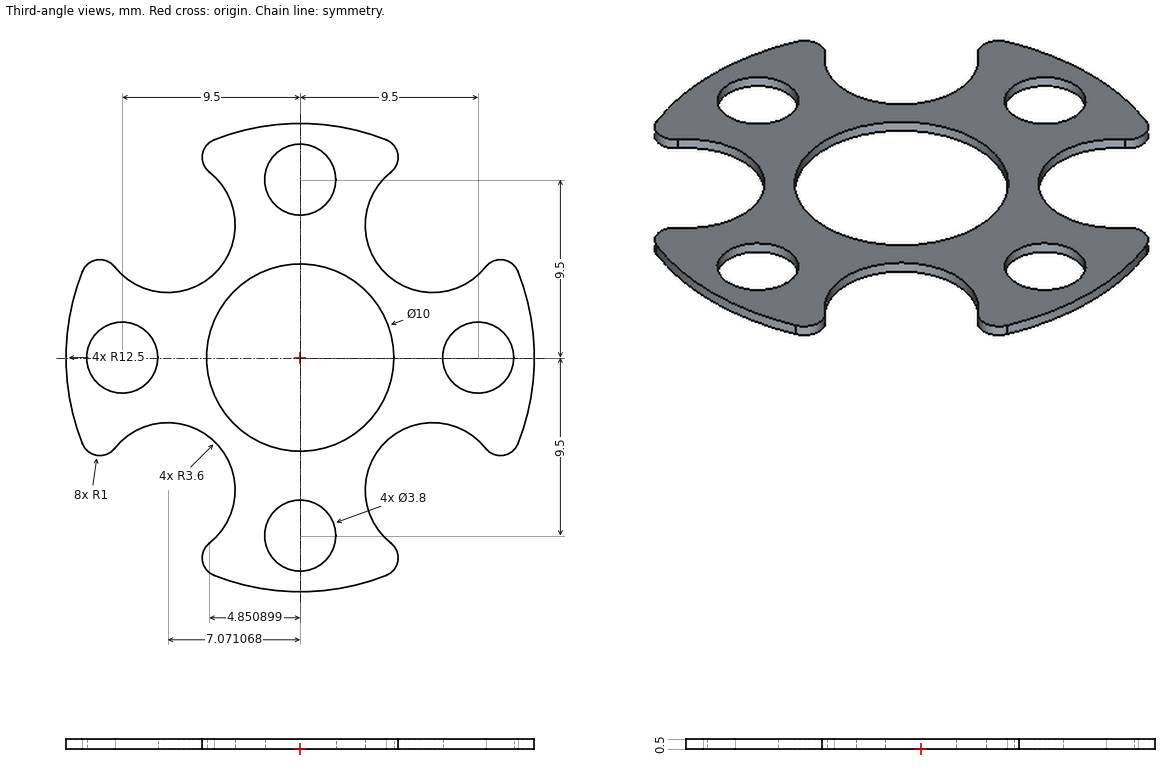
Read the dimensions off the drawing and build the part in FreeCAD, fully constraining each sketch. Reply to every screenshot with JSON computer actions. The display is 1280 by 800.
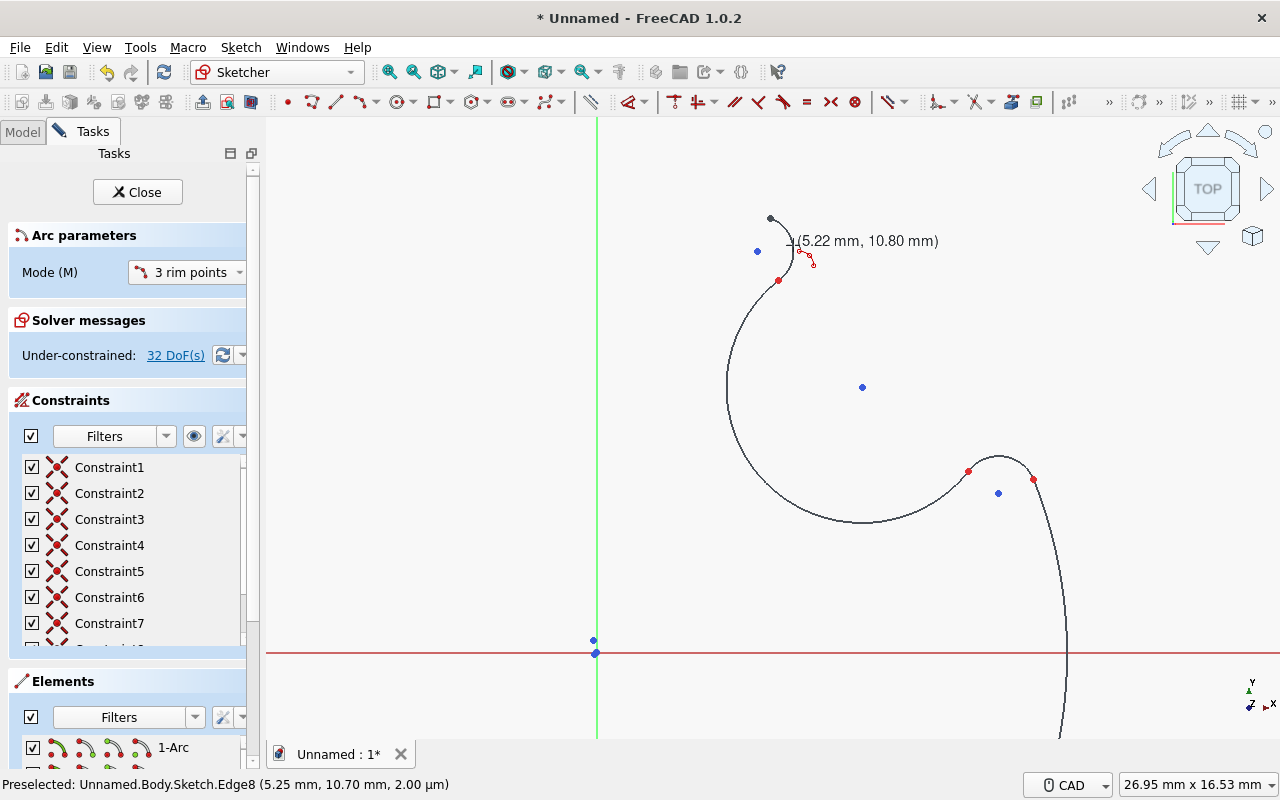
{"action": "left_click", "coordinate": [770, 218]}
{"action": "left_click", "coordinate": [423, 215]}
{"action": "left_click", "coordinate": [632, 184]}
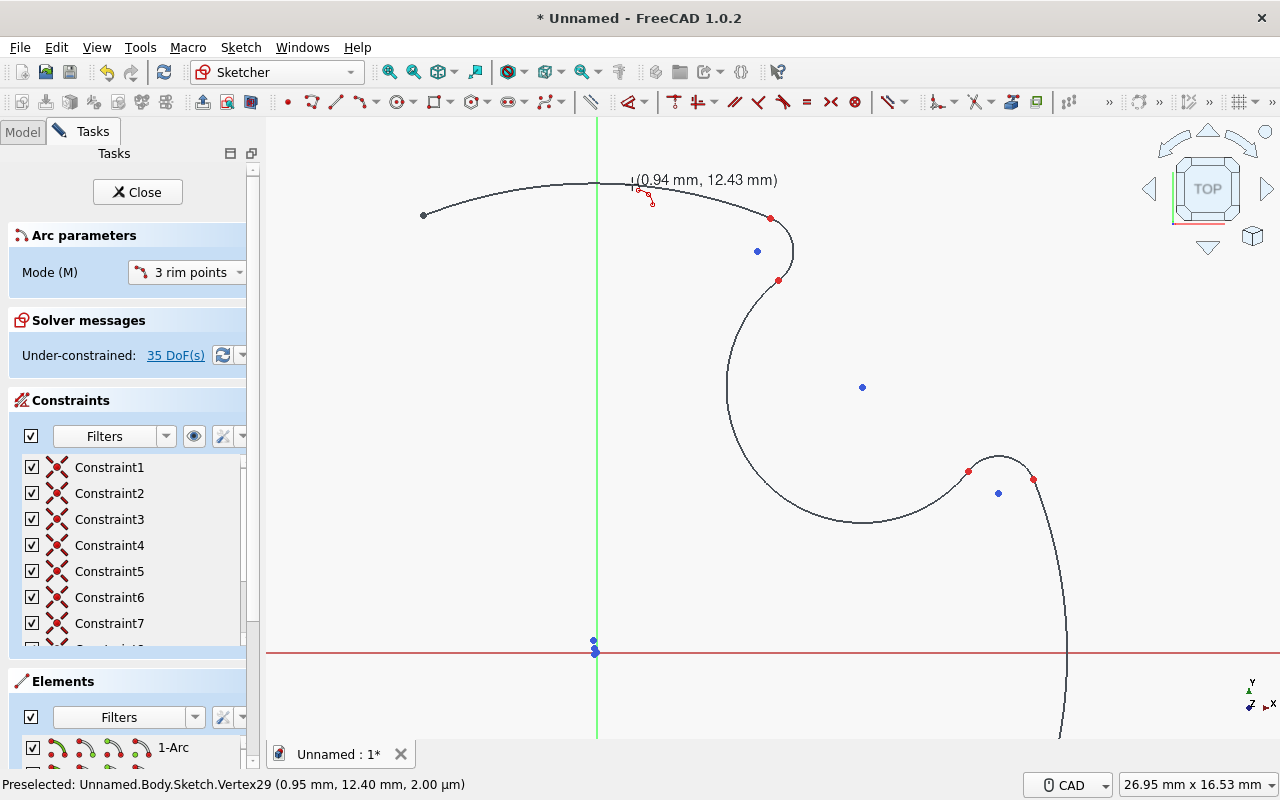
{"action": "left_click", "coordinate": [423, 216]}
{"action": "left_click", "coordinate": [414, 280]}
{"action": "left_click", "coordinate": [400, 245]}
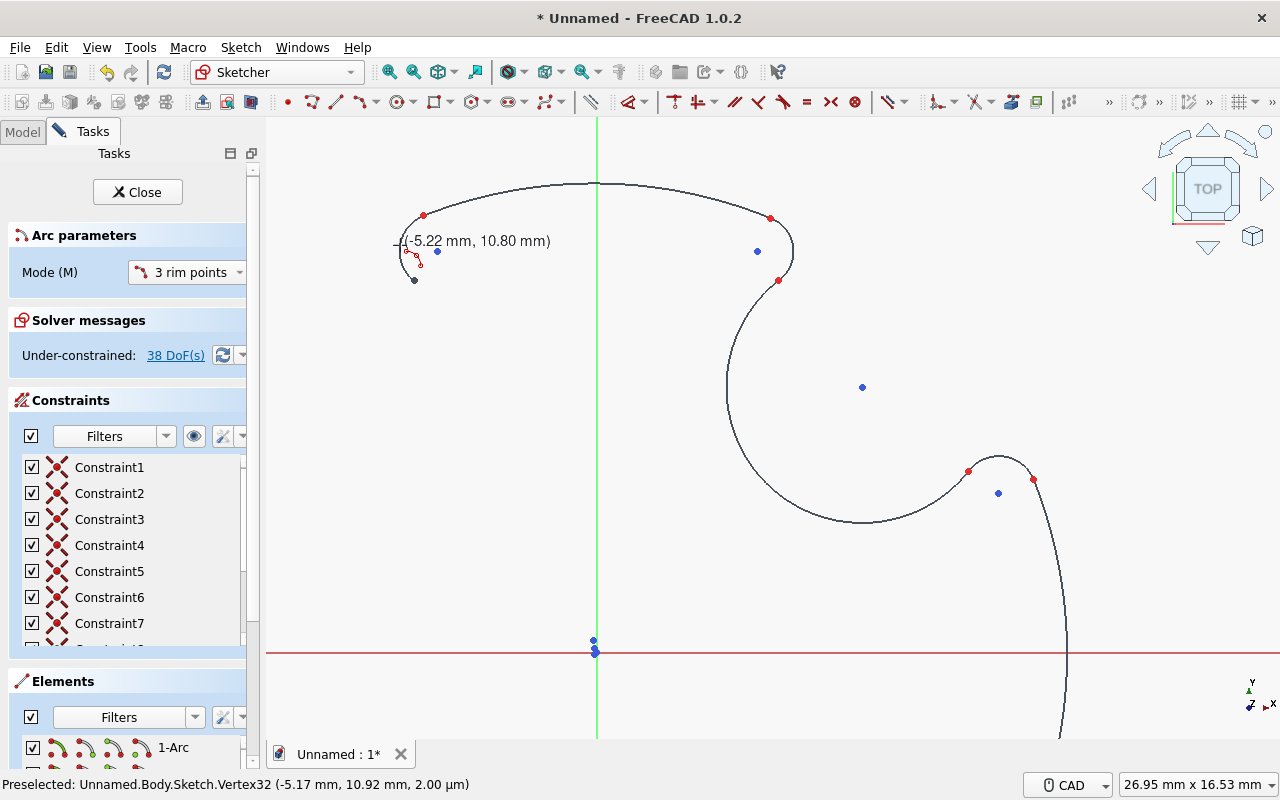
{"action": "left_click", "coordinate": [414, 281]}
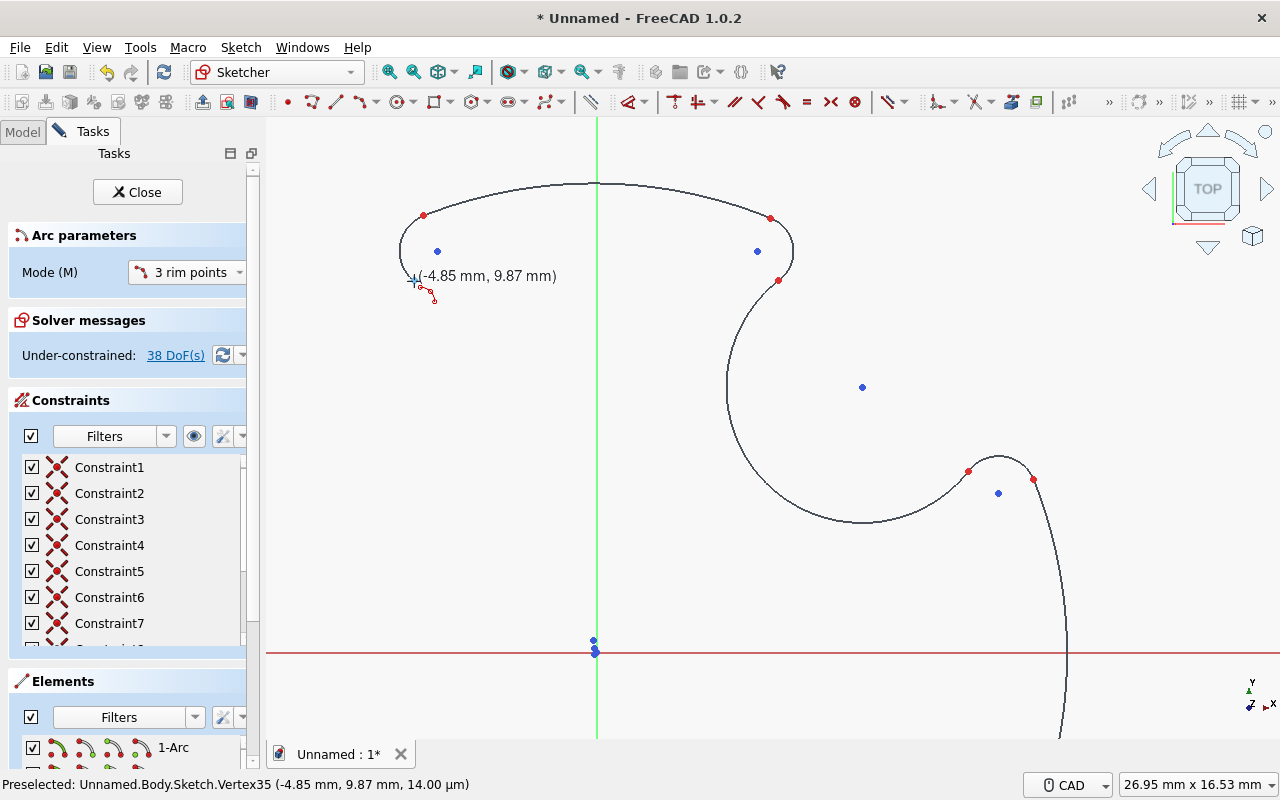
{"action": "scroll", "coordinate": [793, 245], "scroll_direction": "down", "scroll_amount": 4}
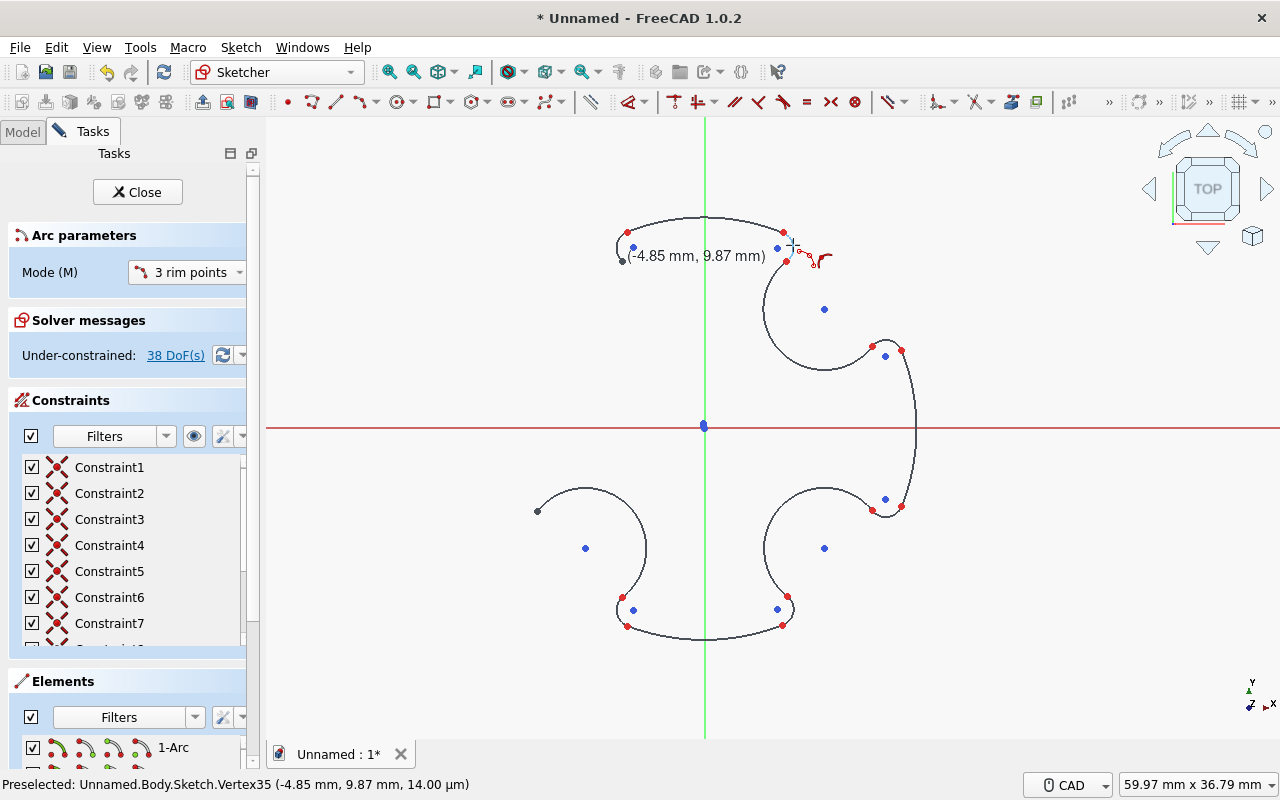
{"action": "left_click", "coordinate": [538, 346]}
{"action": "left_click", "coordinate": [628, 352]}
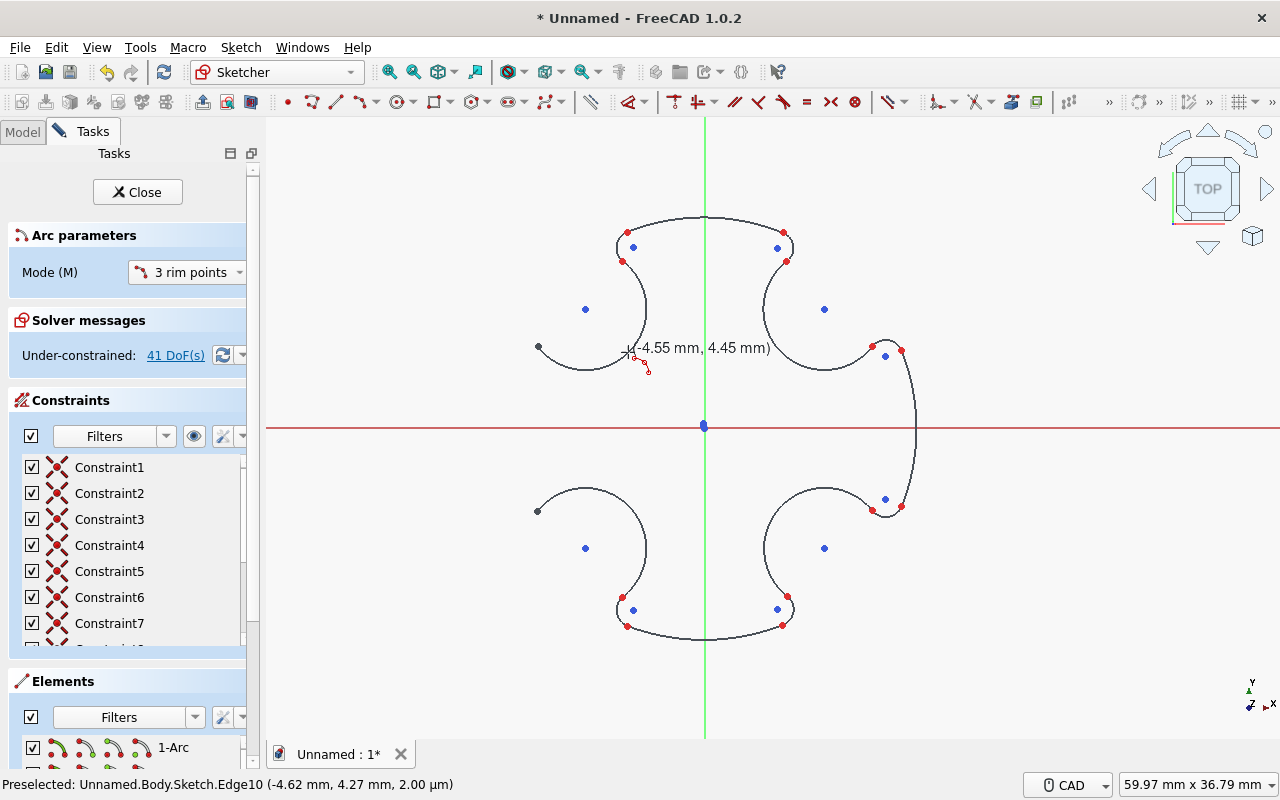
{"action": "left_click", "coordinate": [538, 347]}
{"action": "left_click", "coordinate": [508, 350]}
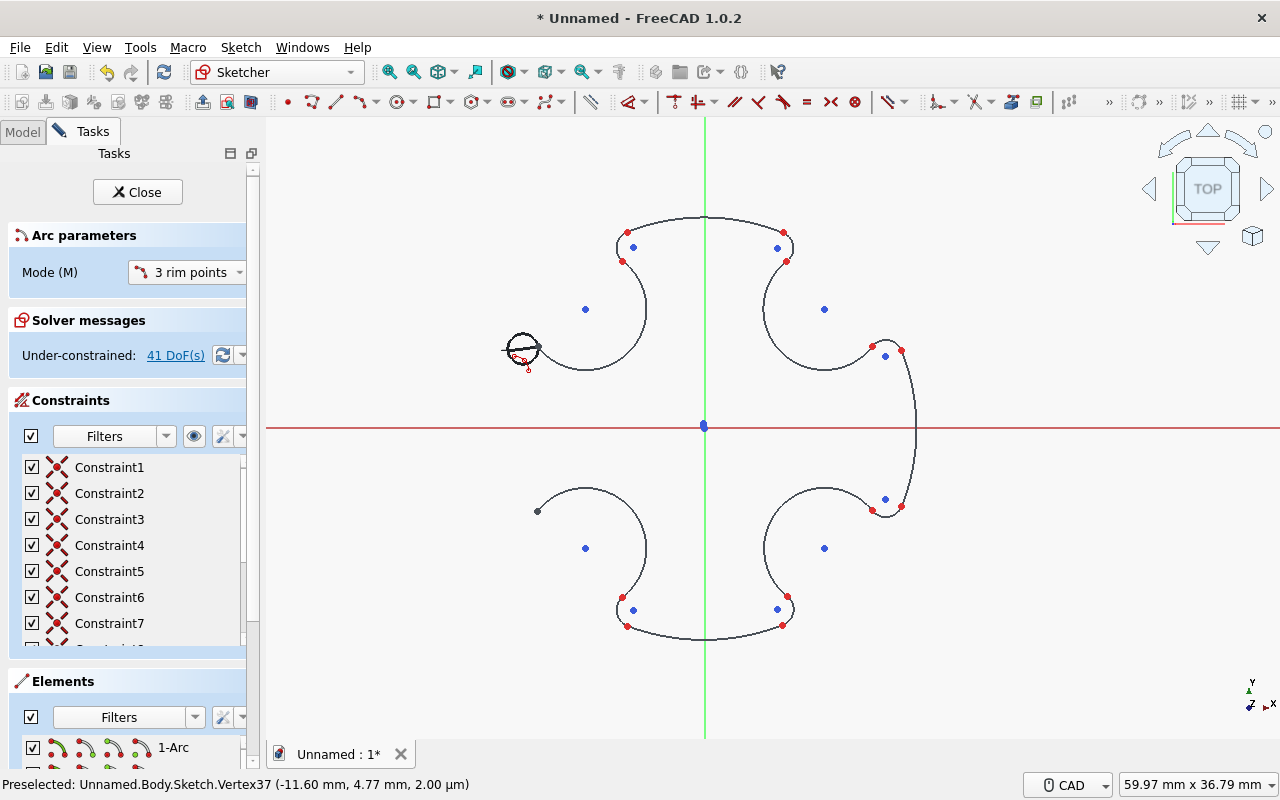
{"action": "scroll", "coordinate": [522, 340], "scroll_direction": "up", "scroll_amount": 4}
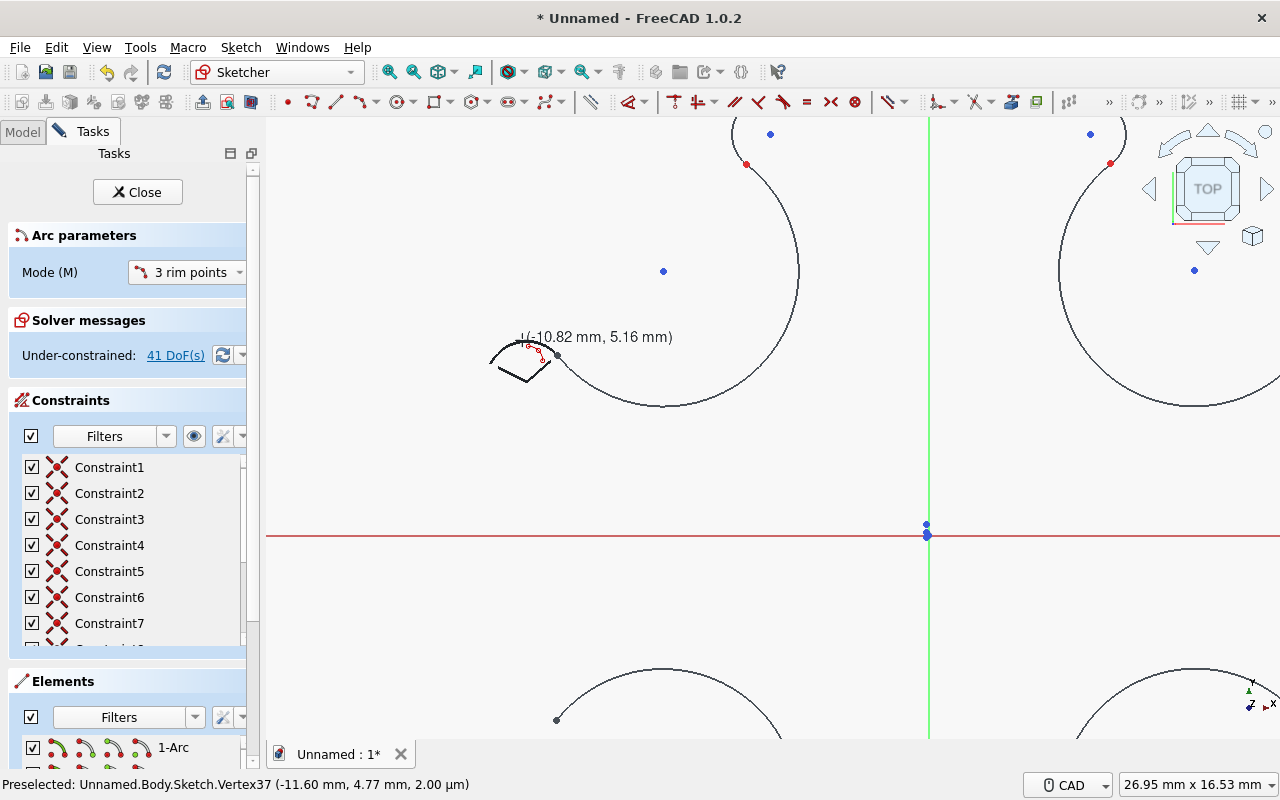
{"action": "left_click", "coordinate": [521, 339]}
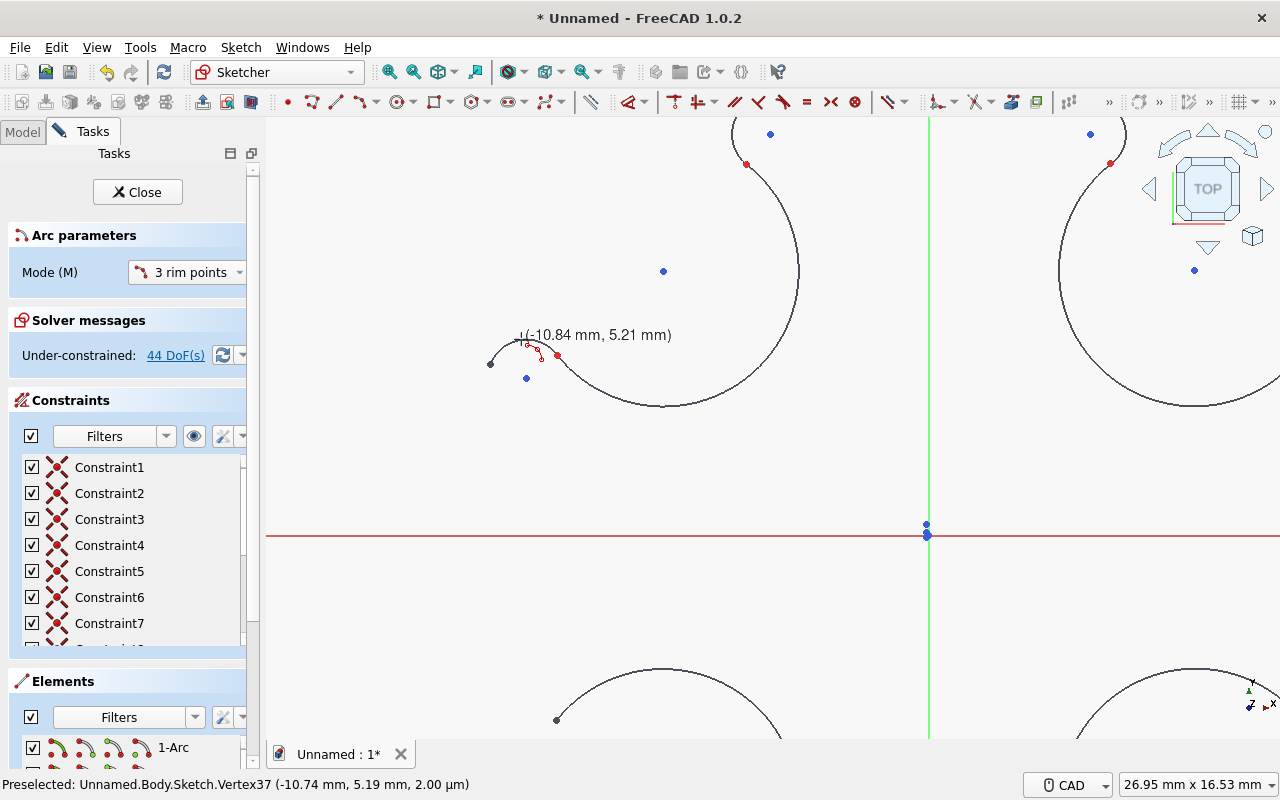
{"action": "left_click", "coordinate": [491, 364]}
{"action": "left_click", "coordinate": [492, 709]}
{"action": "left_click", "coordinate": [460, 501]}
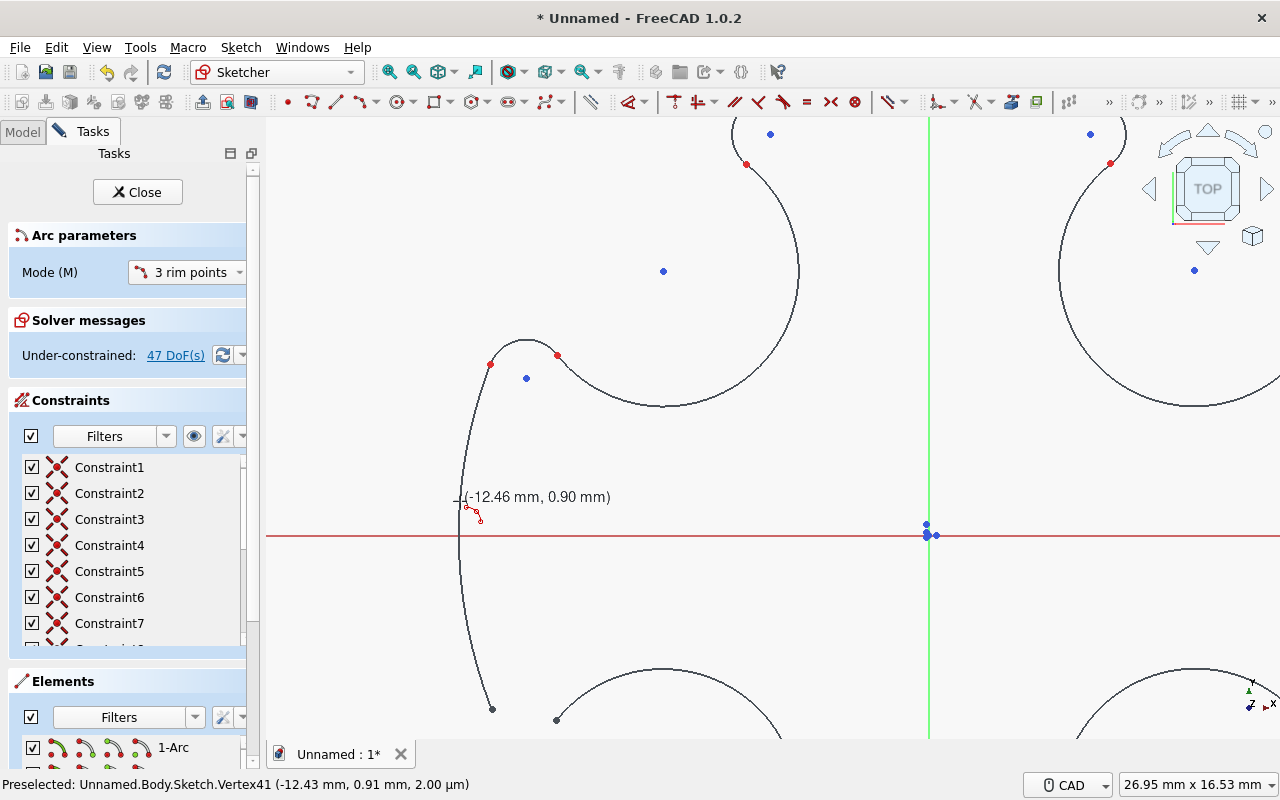
{"action": "left_click", "coordinate": [492, 710]}